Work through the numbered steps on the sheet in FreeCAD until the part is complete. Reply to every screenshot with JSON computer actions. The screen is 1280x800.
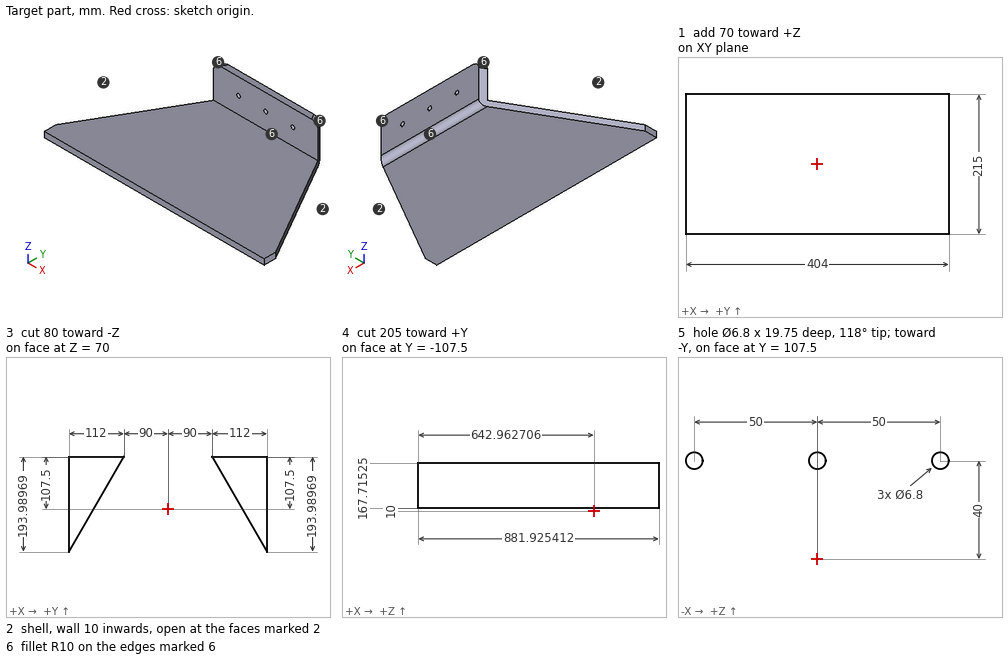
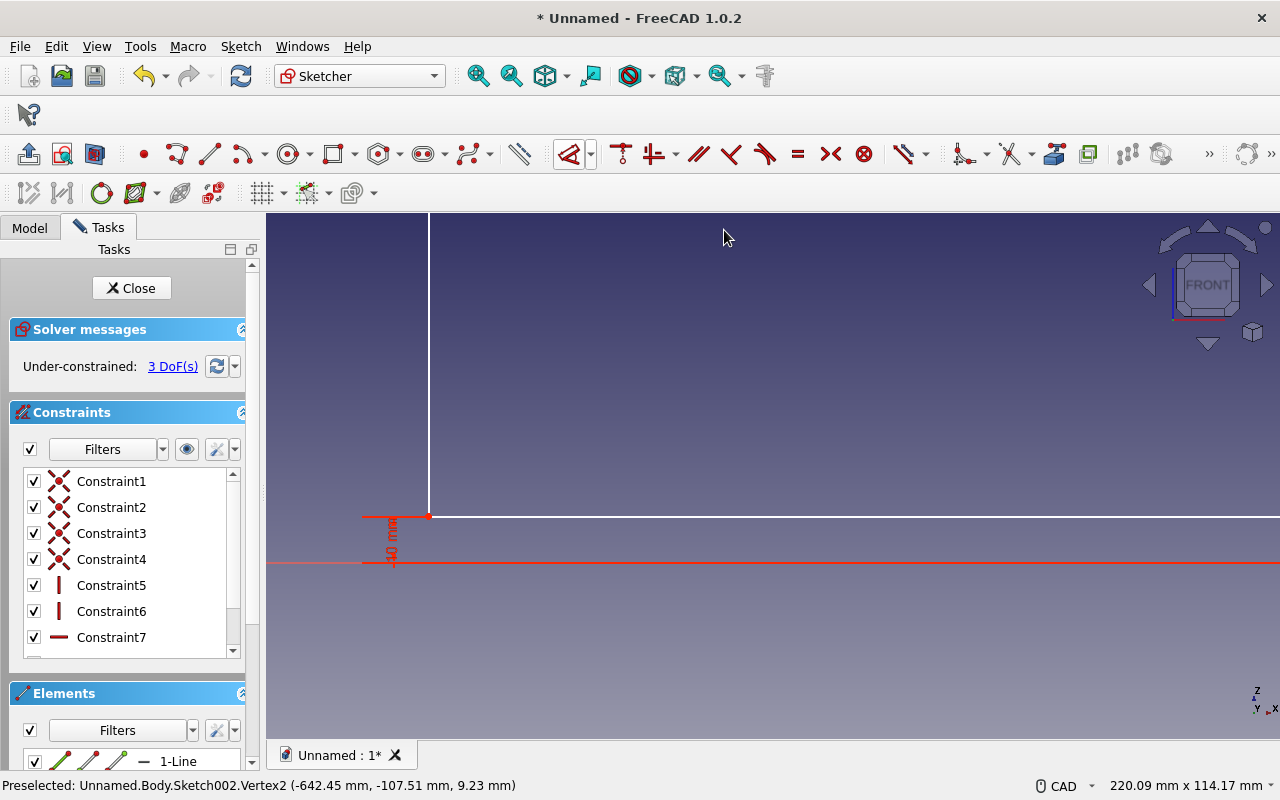
{"action": "scroll", "coordinate": [430, 526], "scroll_direction": "down", "scroll_amount": 10}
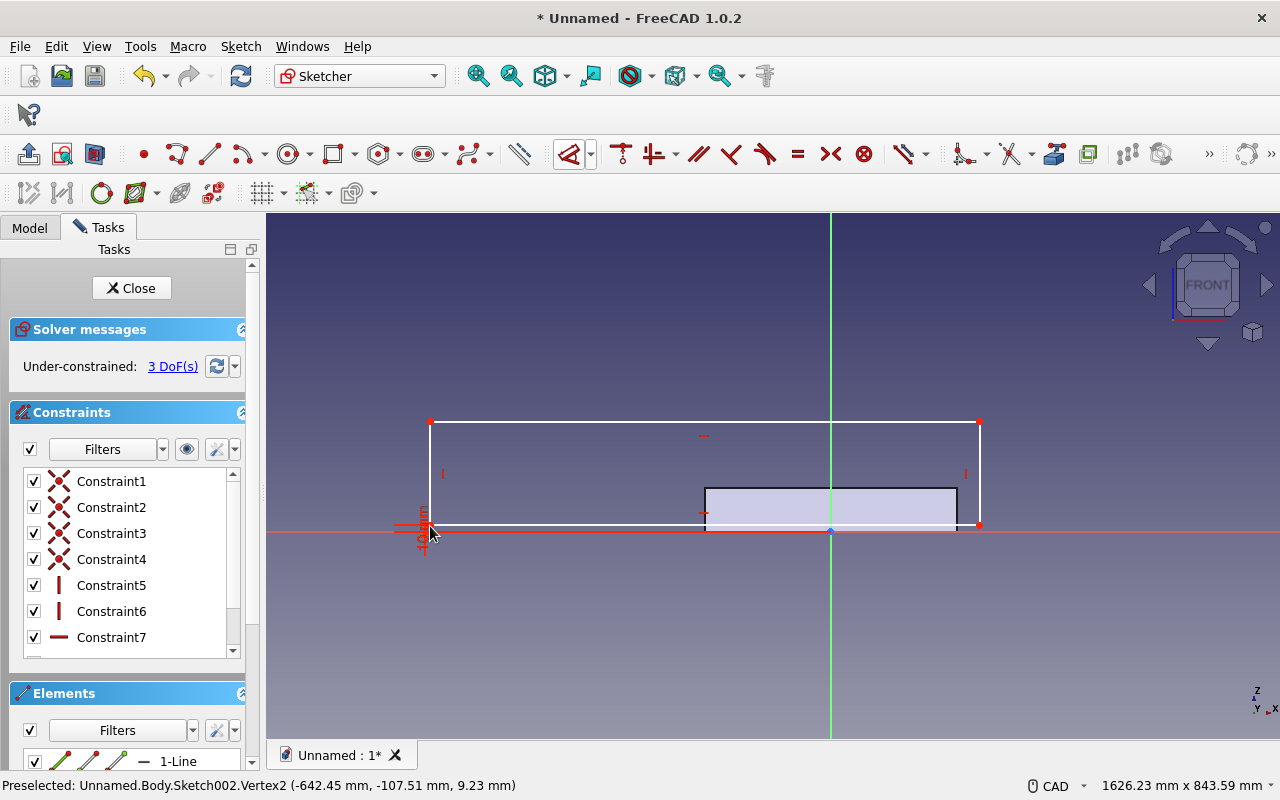
{"action": "left_click", "coordinate": [430, 494]}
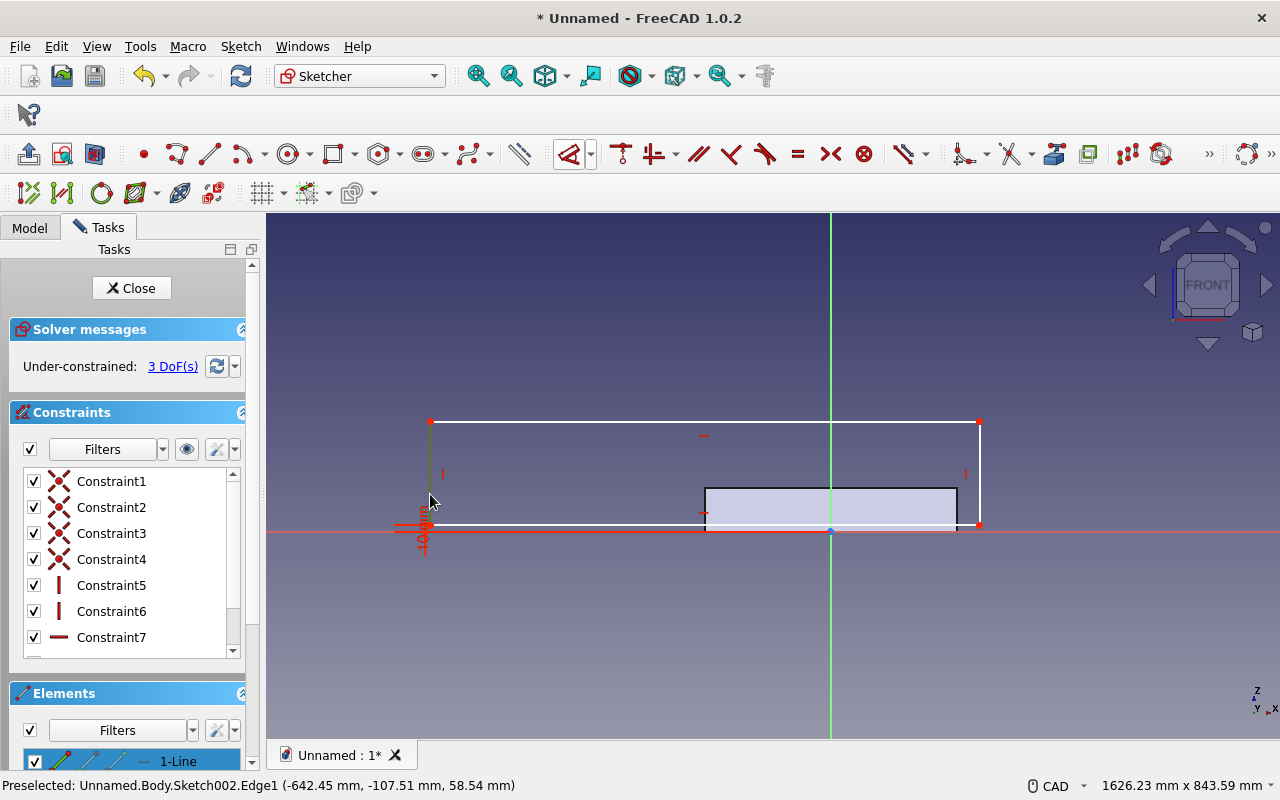
{"action": "left_click", "coordinate": [590, 154]}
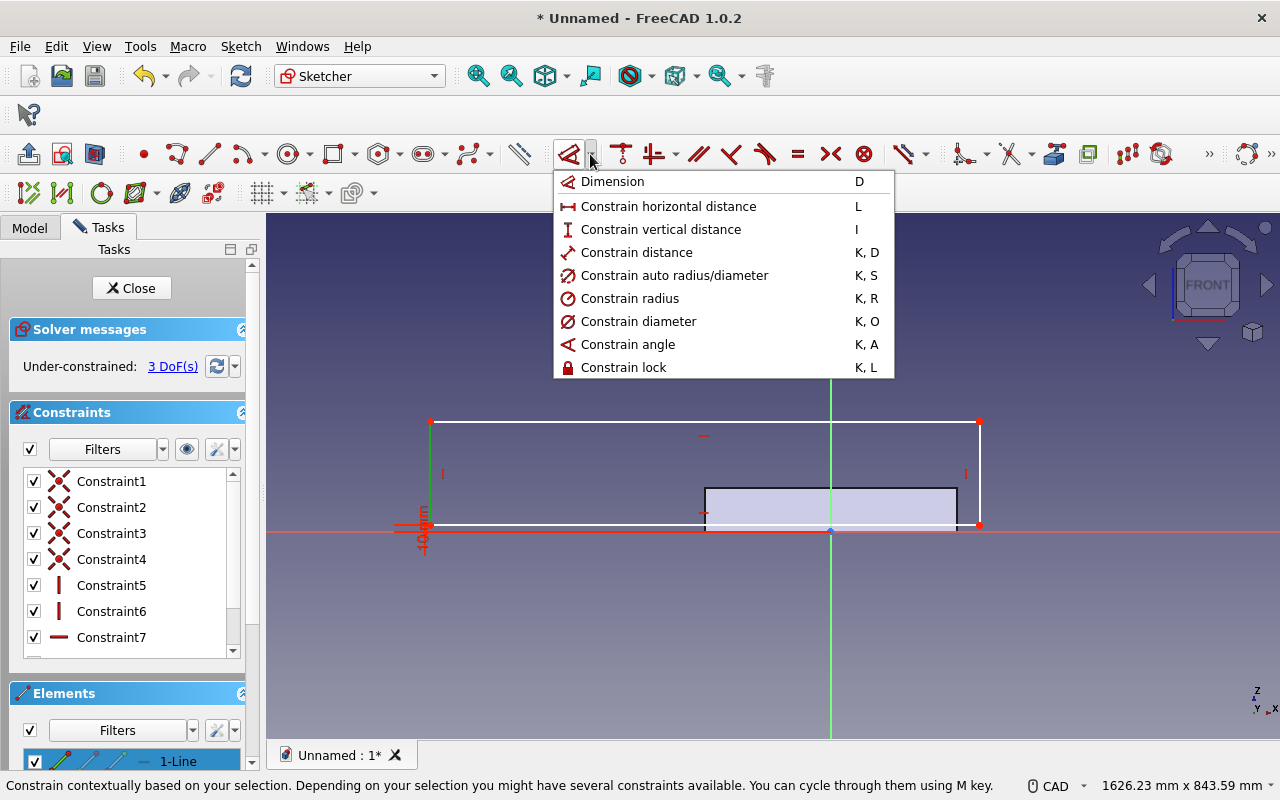
{"action": "left_click", "coordinate": [724, 230]}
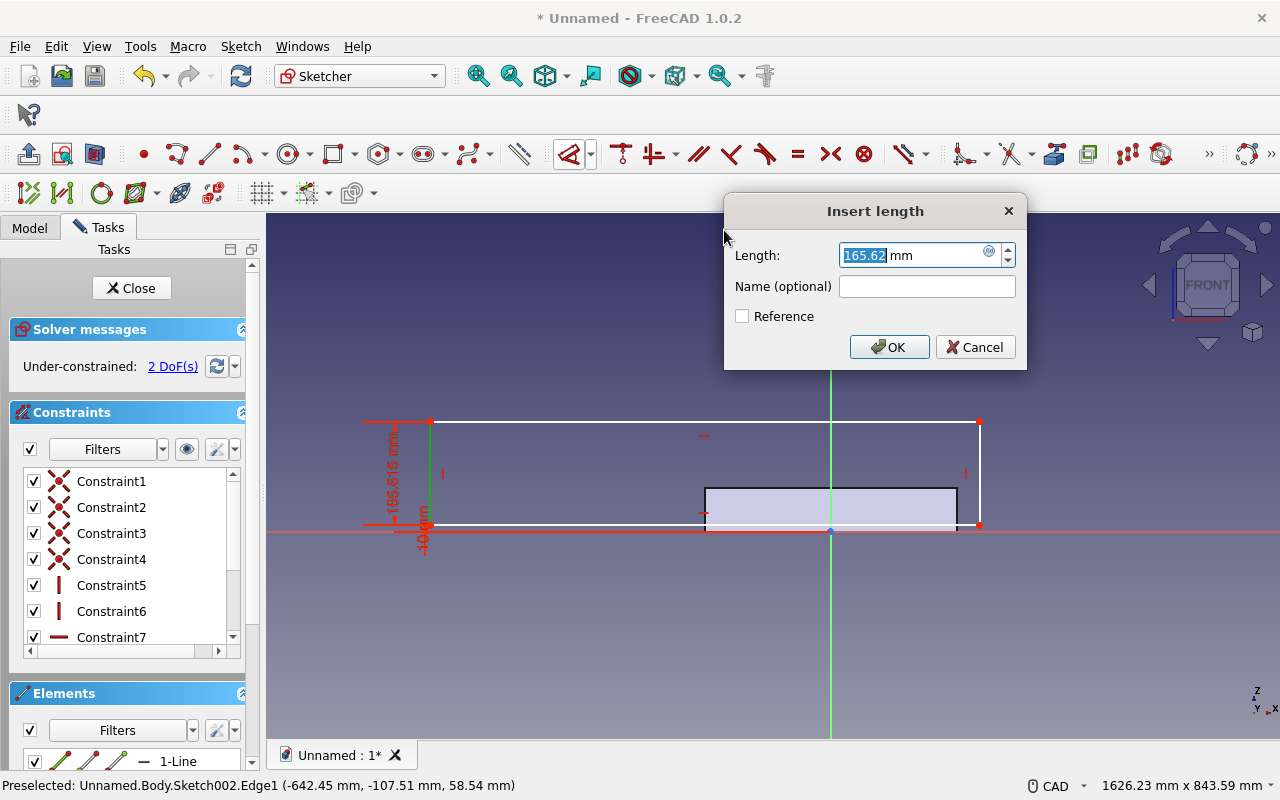
{"action": "type", "text": "167.71525"}
{"action": "key", "text": "Return"}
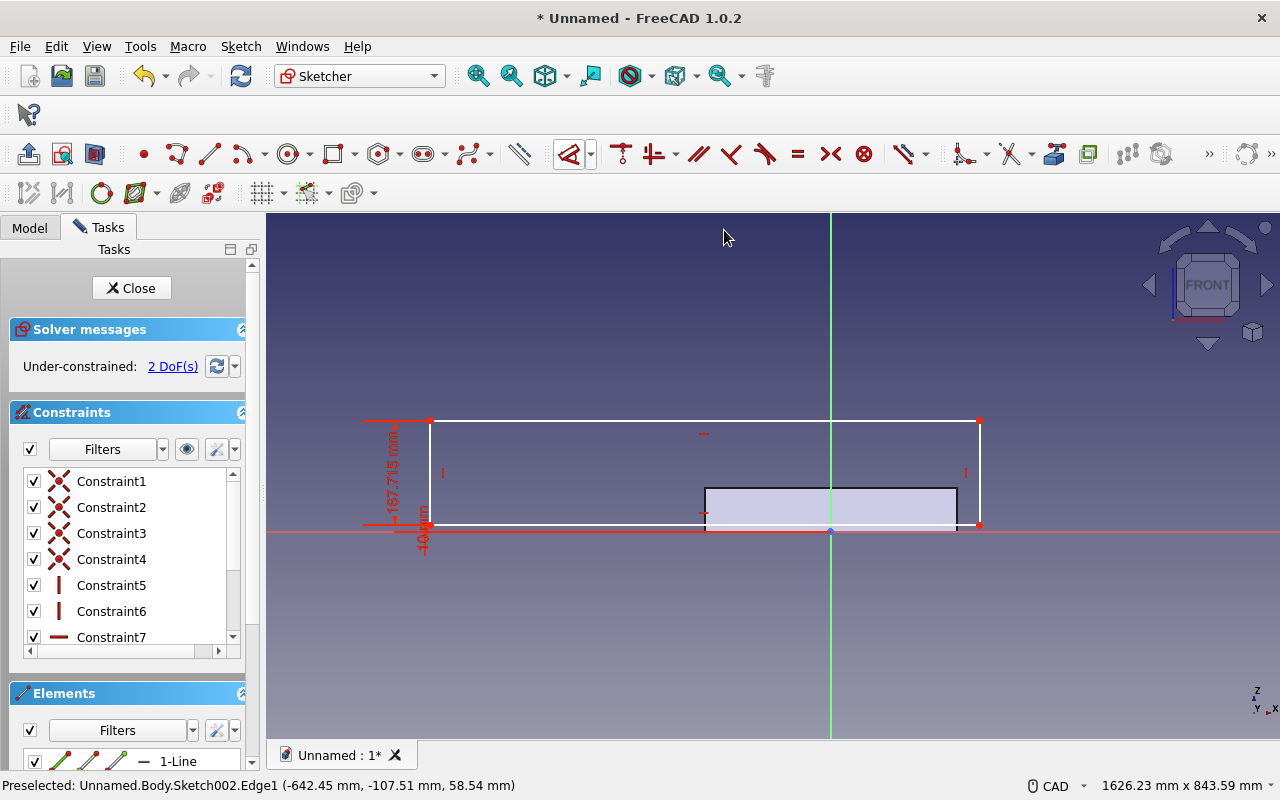
{"action": "scroll", "coordinate": [595, 525], "scroll_direction": "up", "scroll_amount": 4}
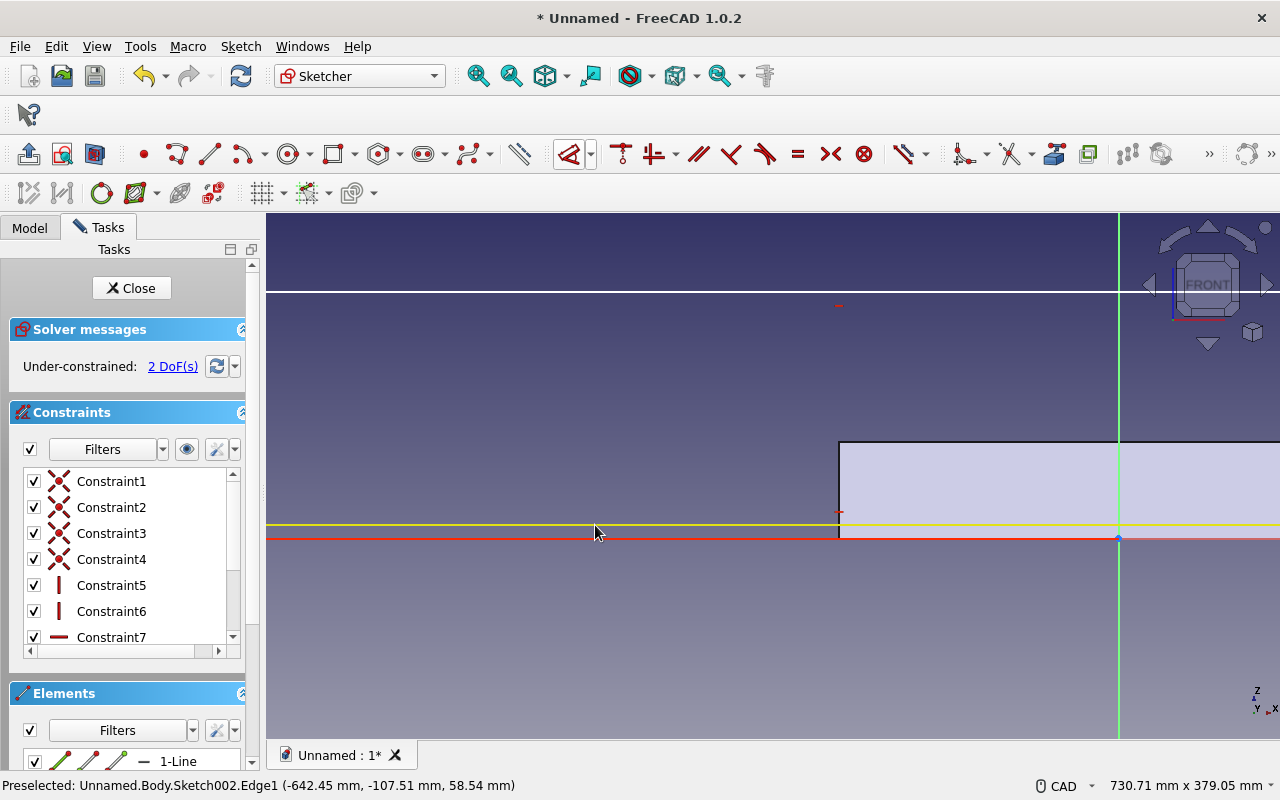
{"action": "left_click", "coordinate": [594, 525]}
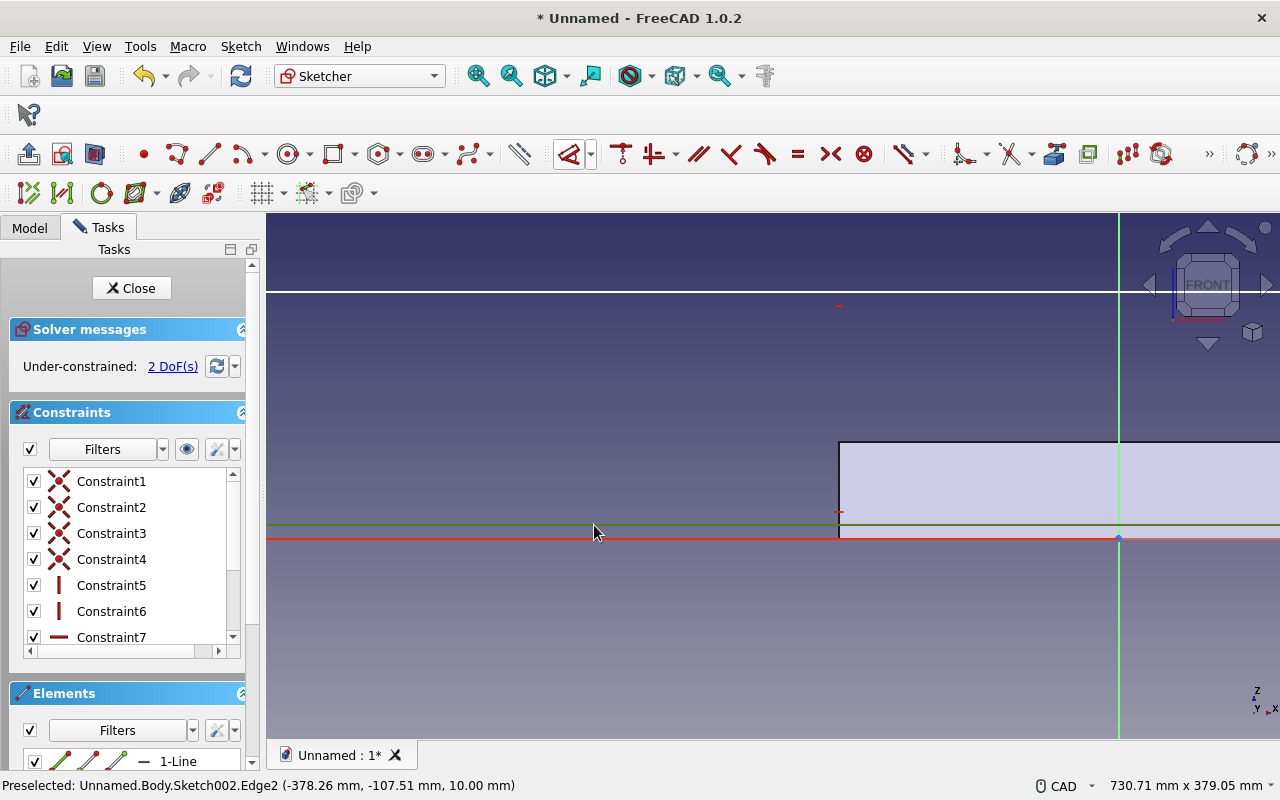
{"action": "key", "text": "l"}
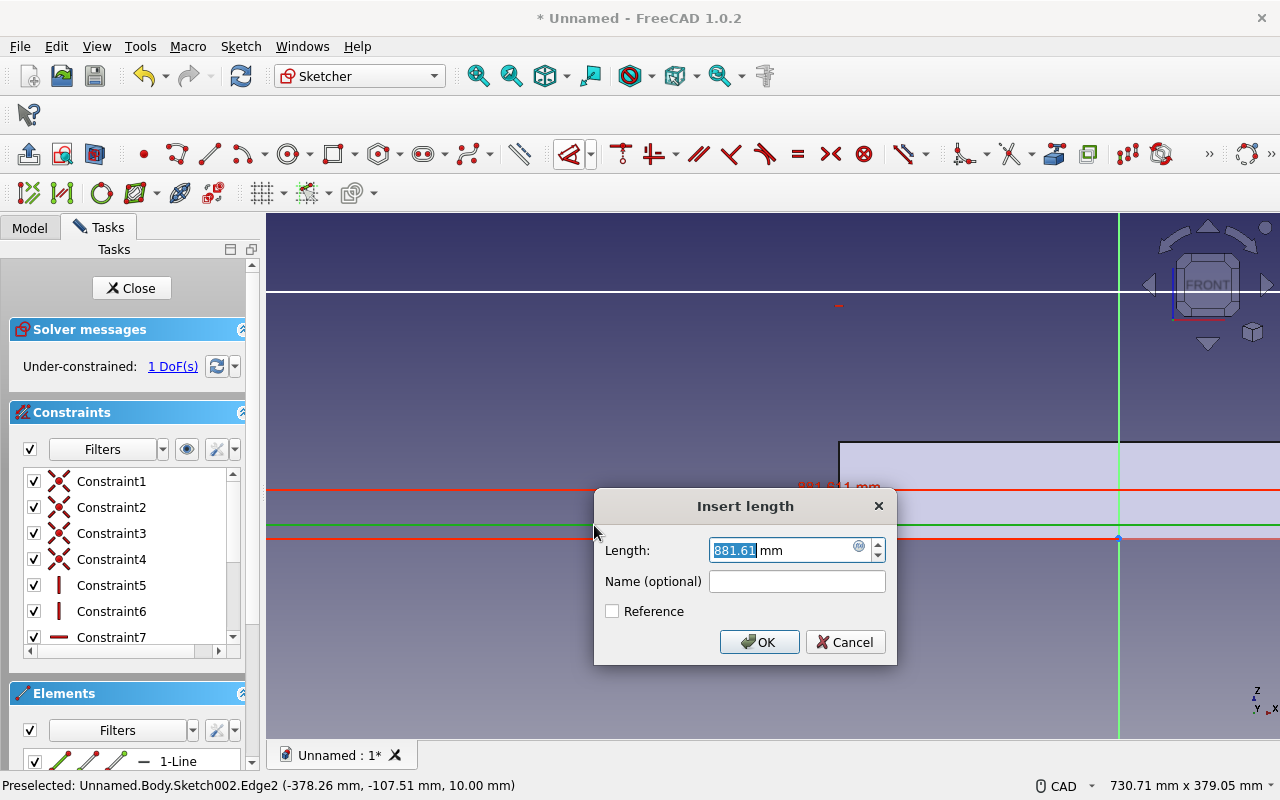
{"action": "type", "text": "881.925412"}
{"action": "key", "text": "Return"}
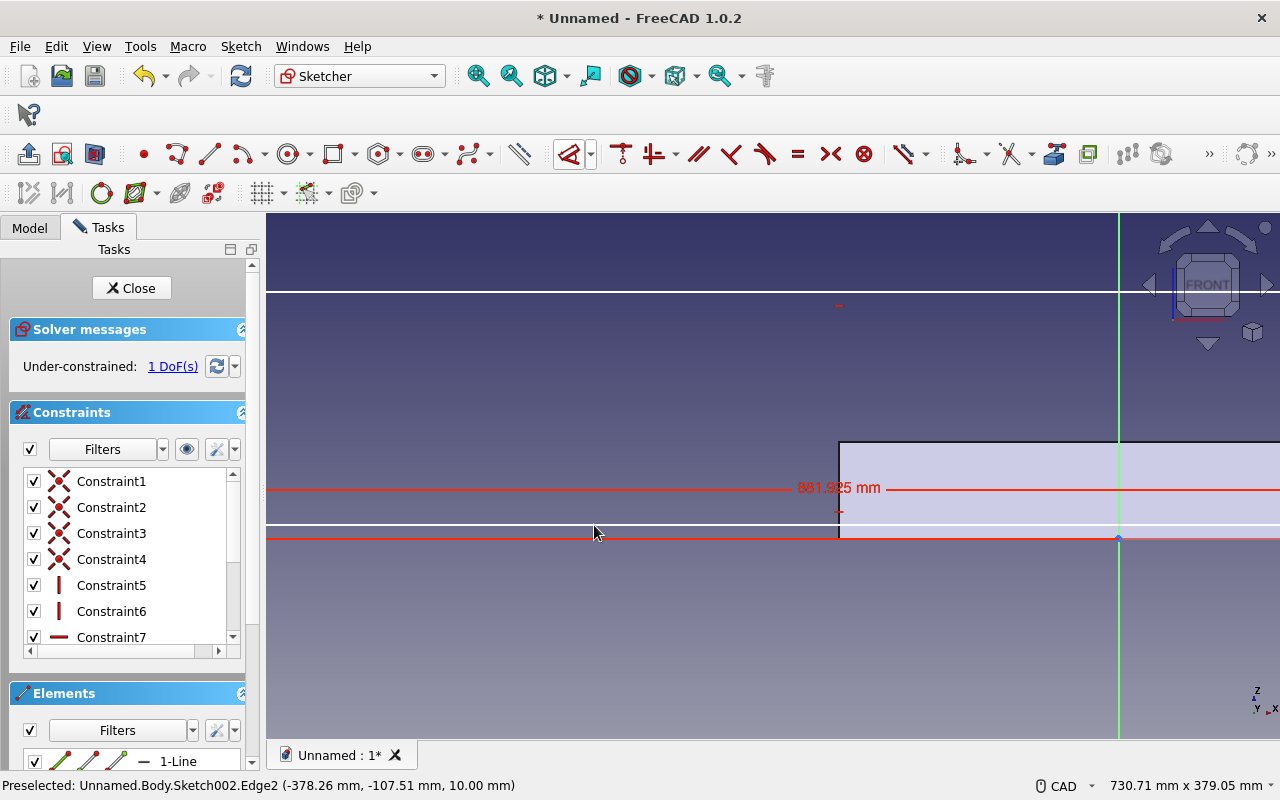
{"action": "scroll", "coordinate": [595, 525], "scroll_direction": "down", "scroll_amount": 4}